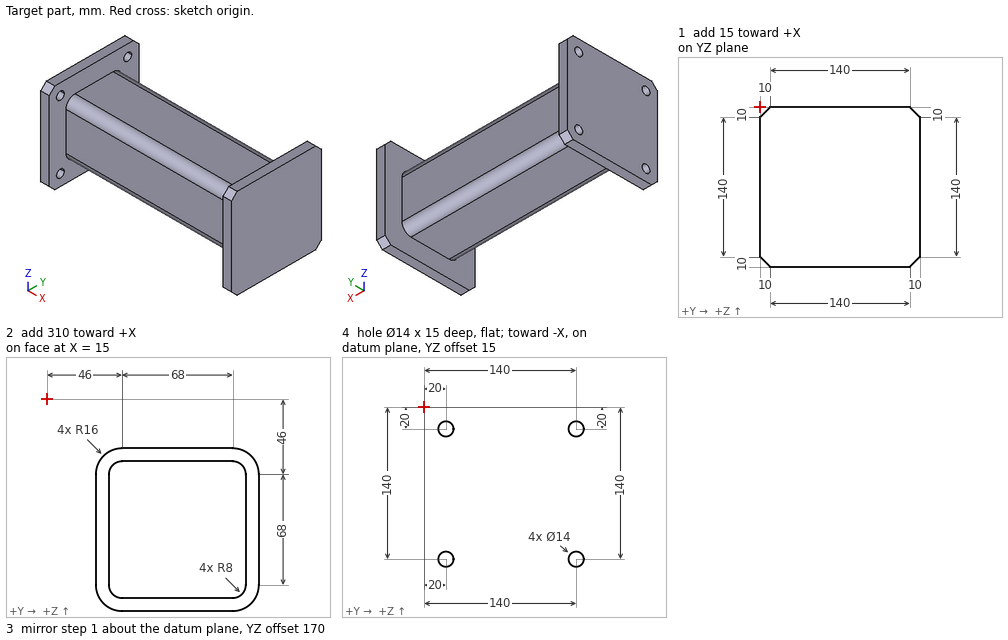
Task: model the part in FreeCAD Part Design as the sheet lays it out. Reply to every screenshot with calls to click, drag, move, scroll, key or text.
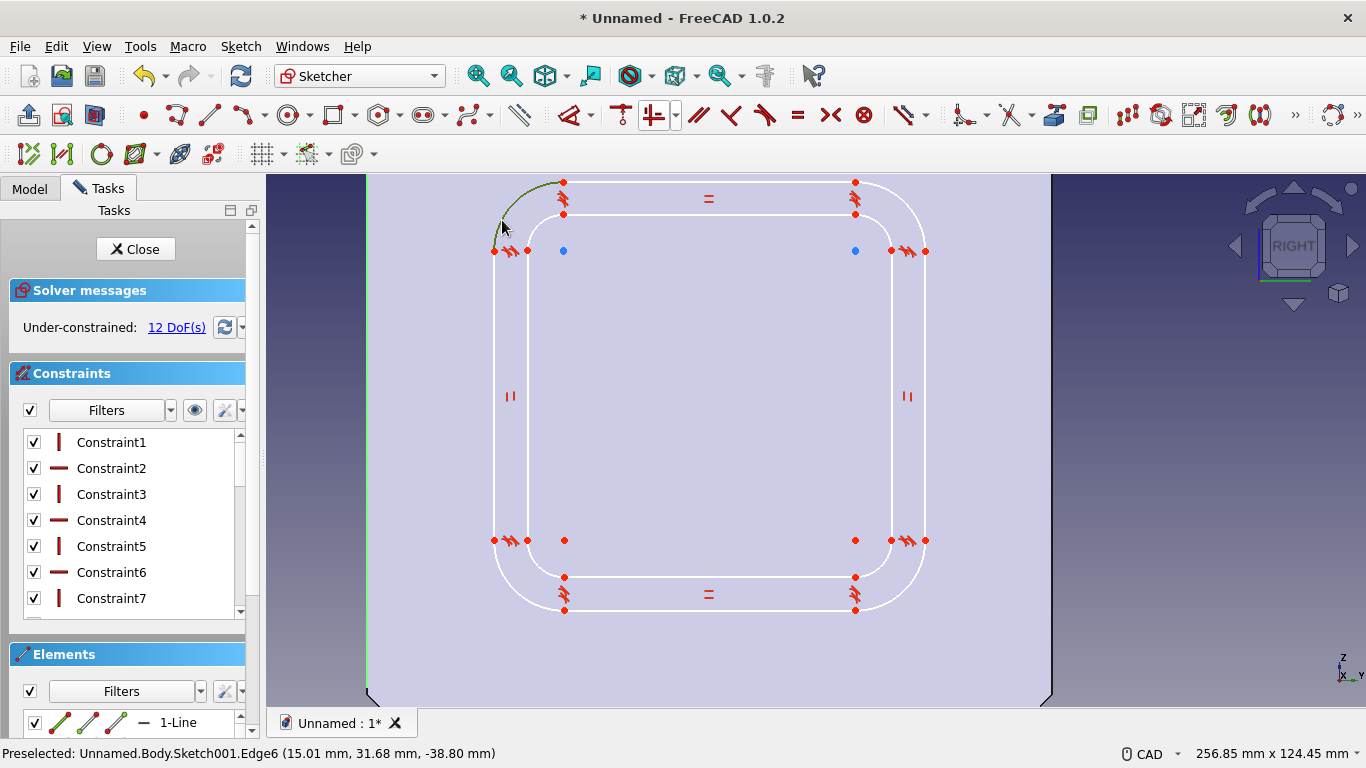
click(547, 219)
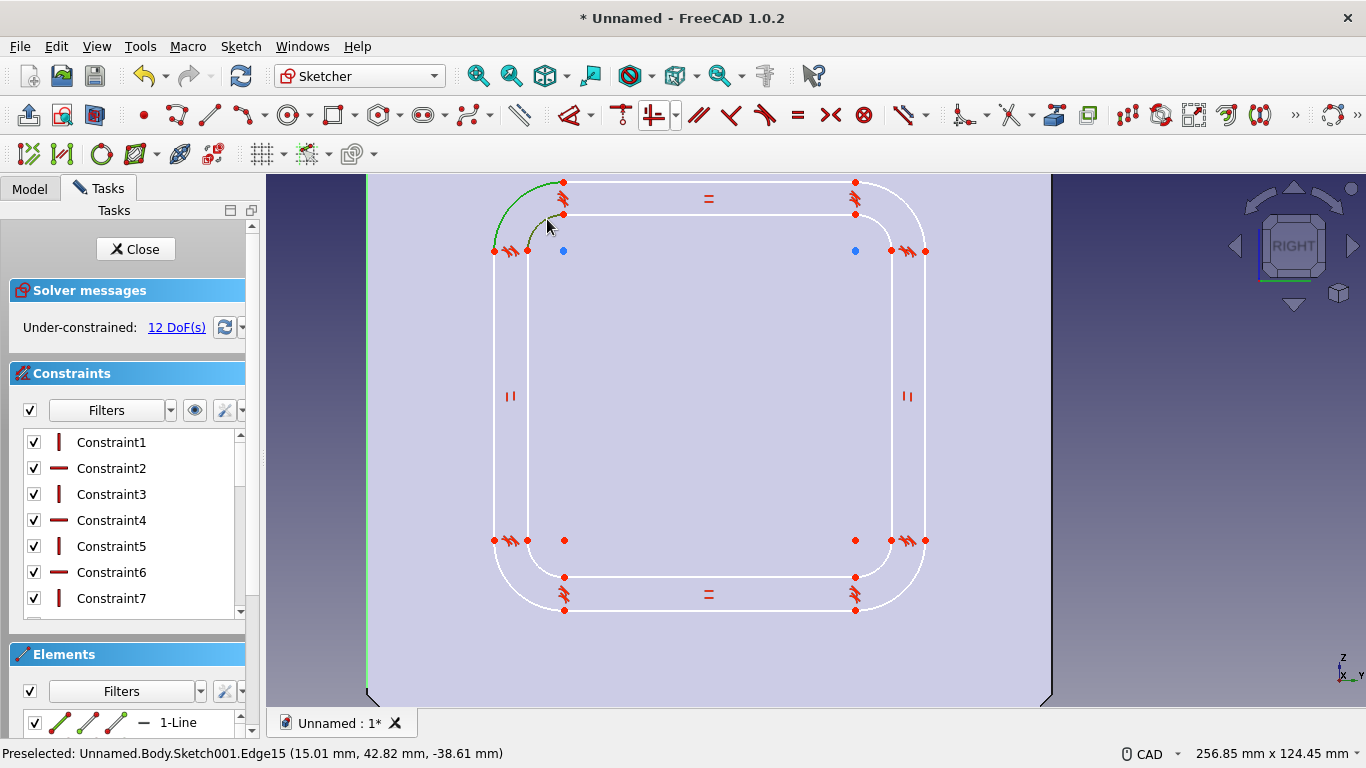
key(c)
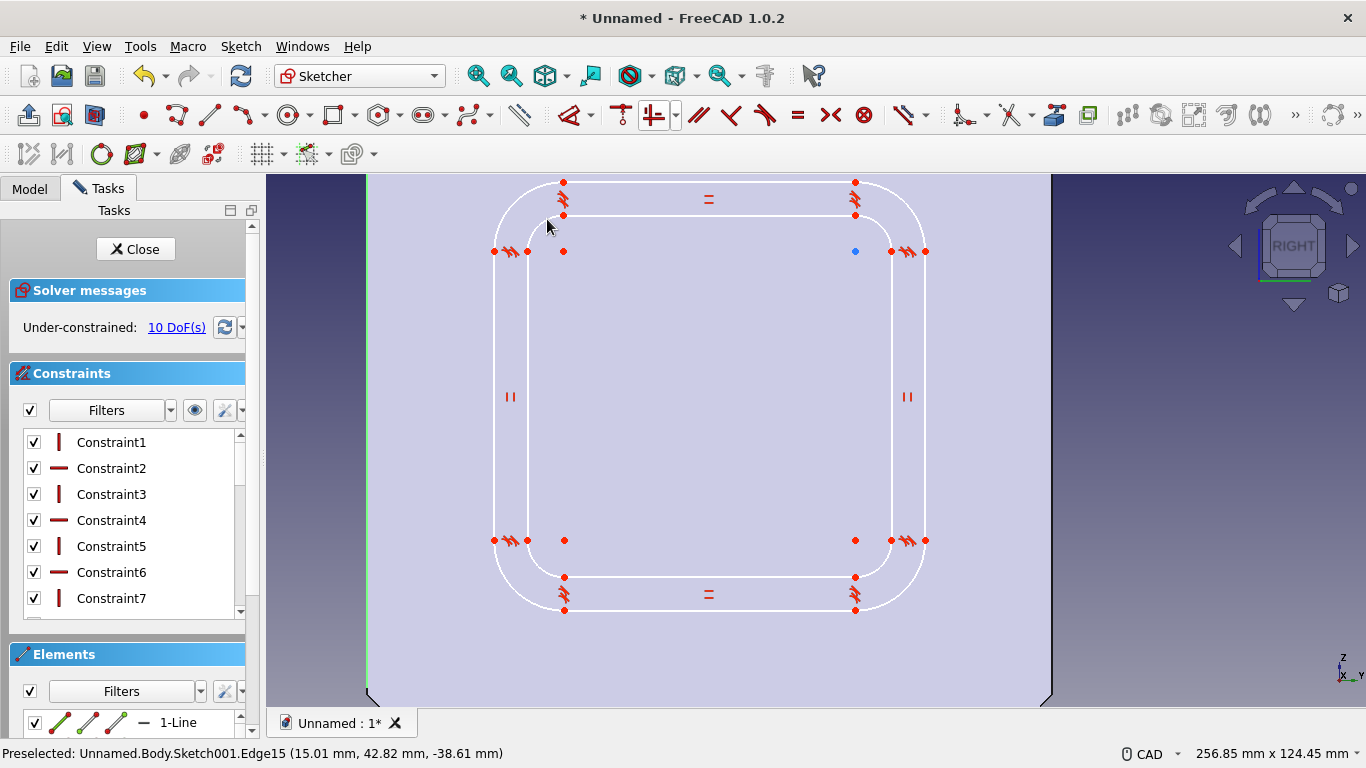
click(918, 220)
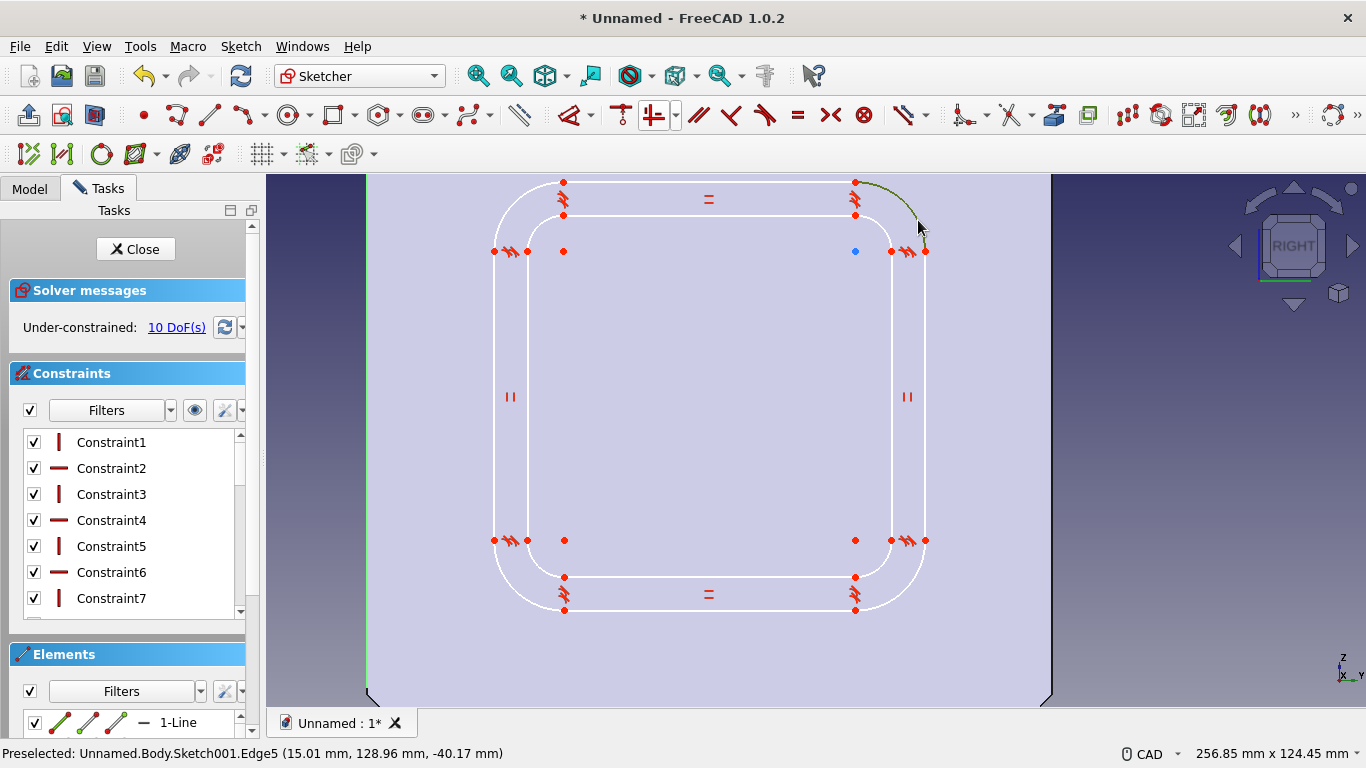
click(502, 220)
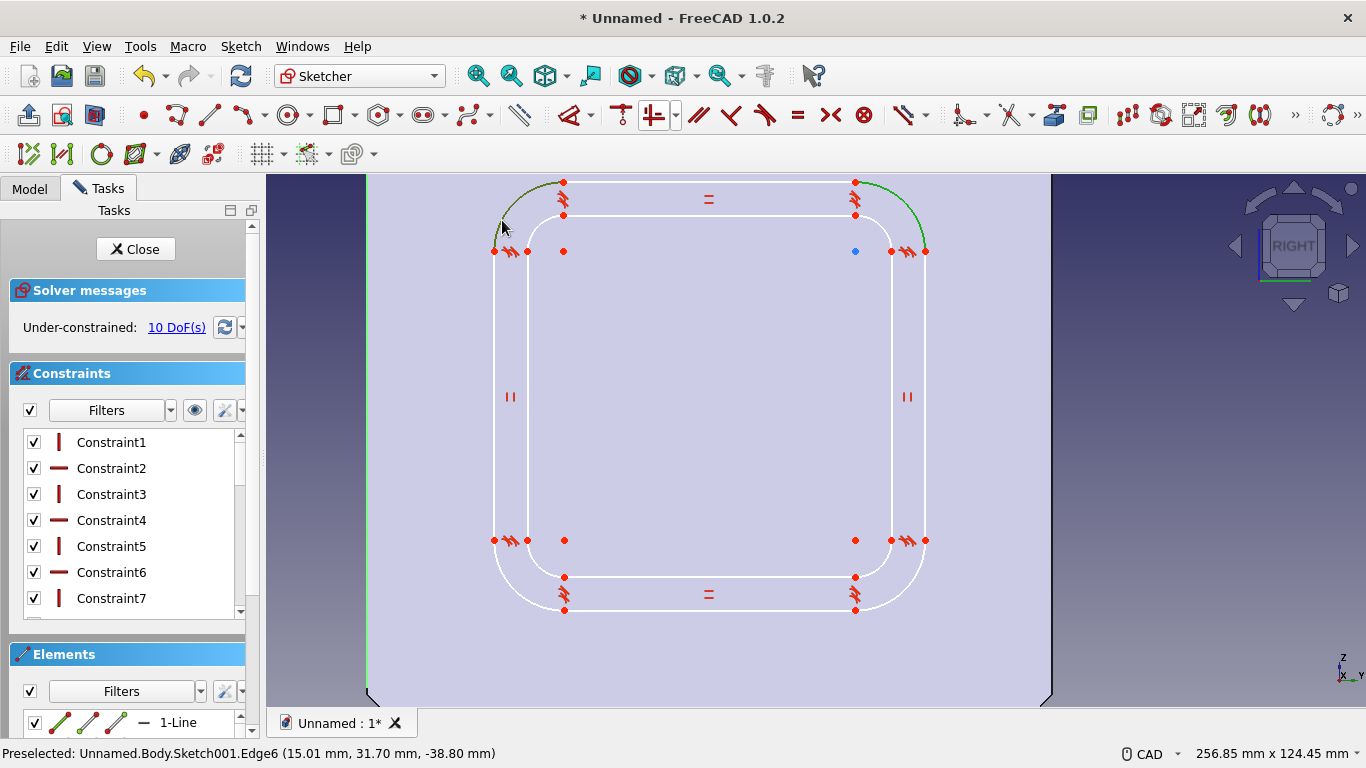
click(502, 573)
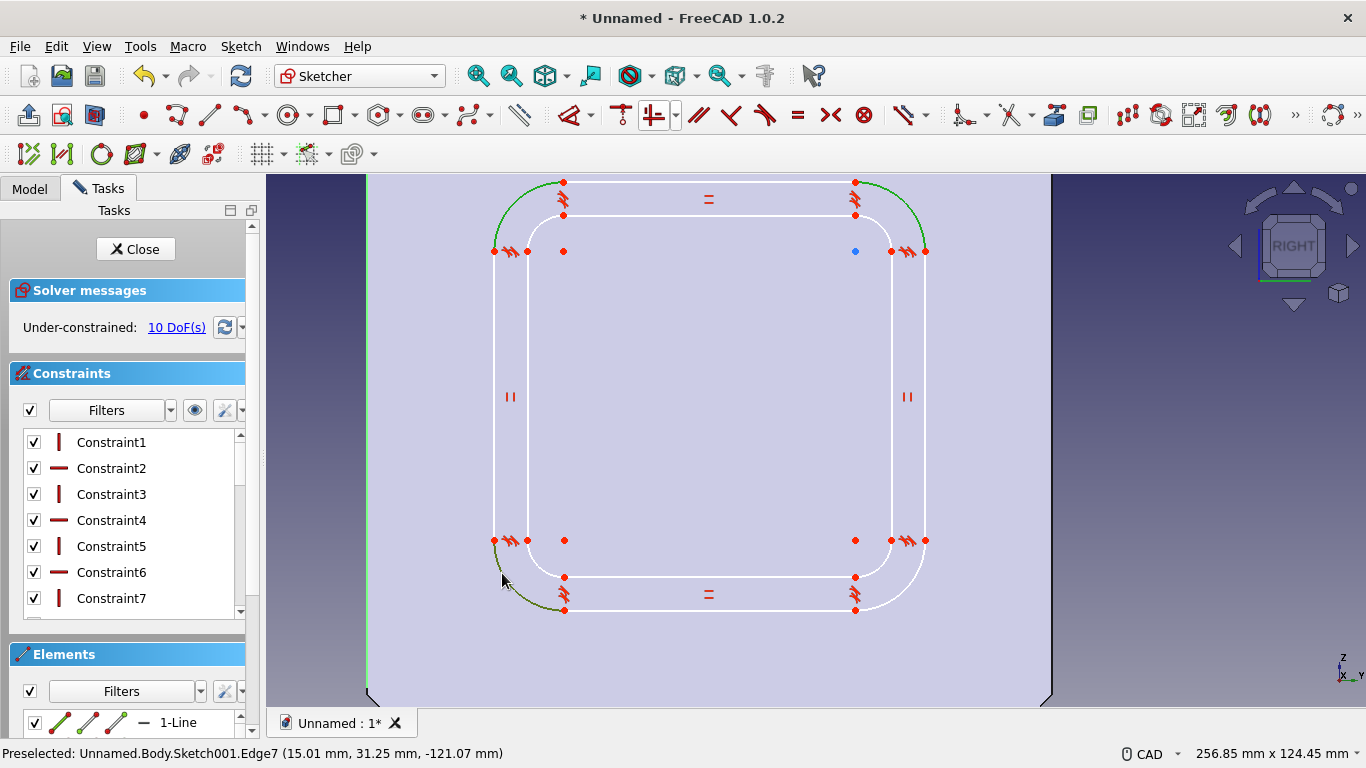
click(887, 603)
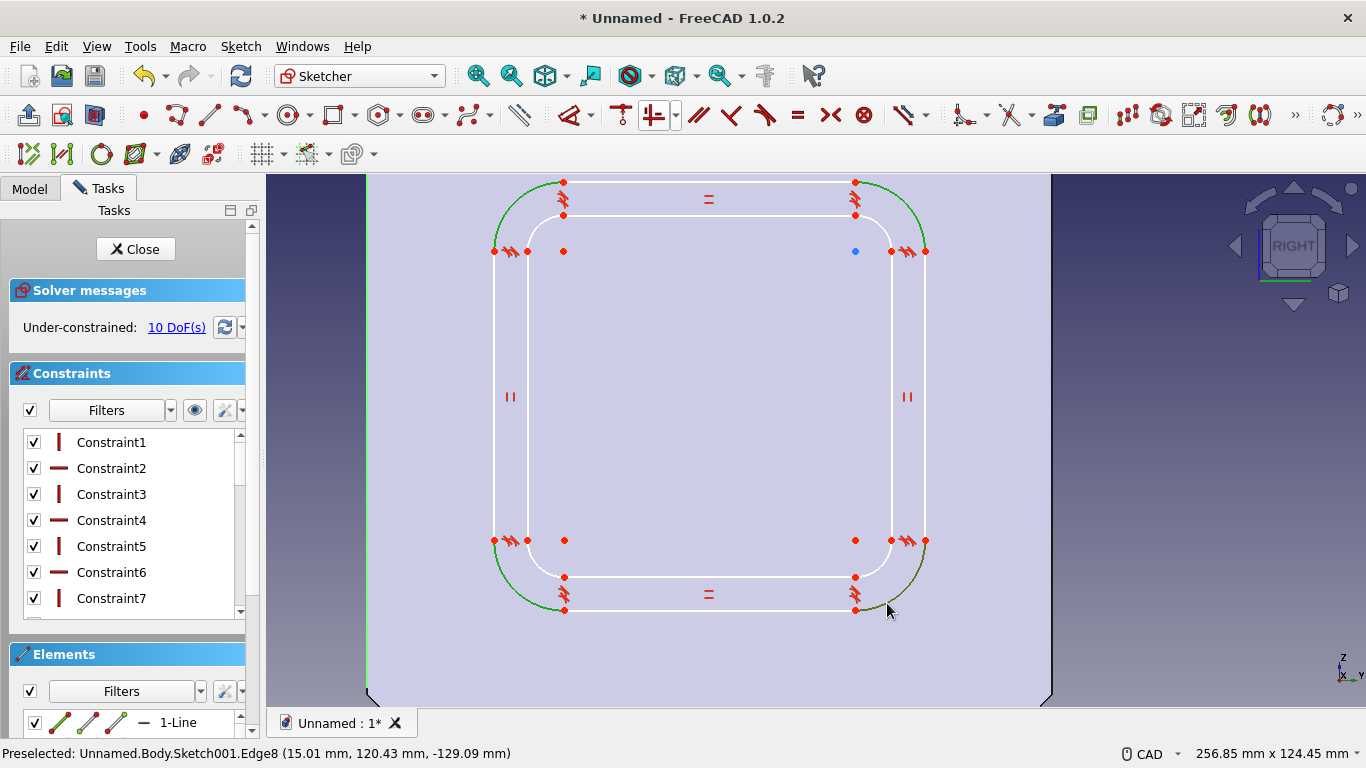
click(798, 116)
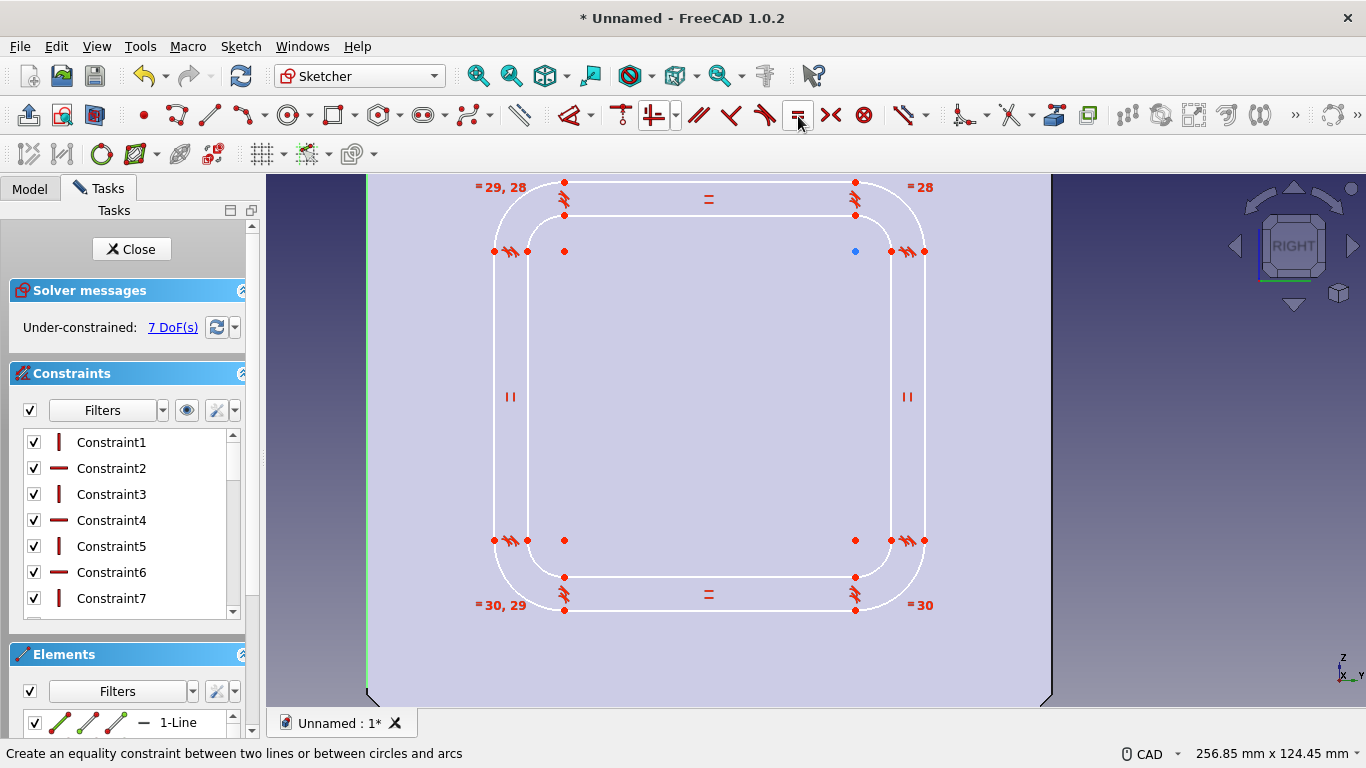
click(872, 573)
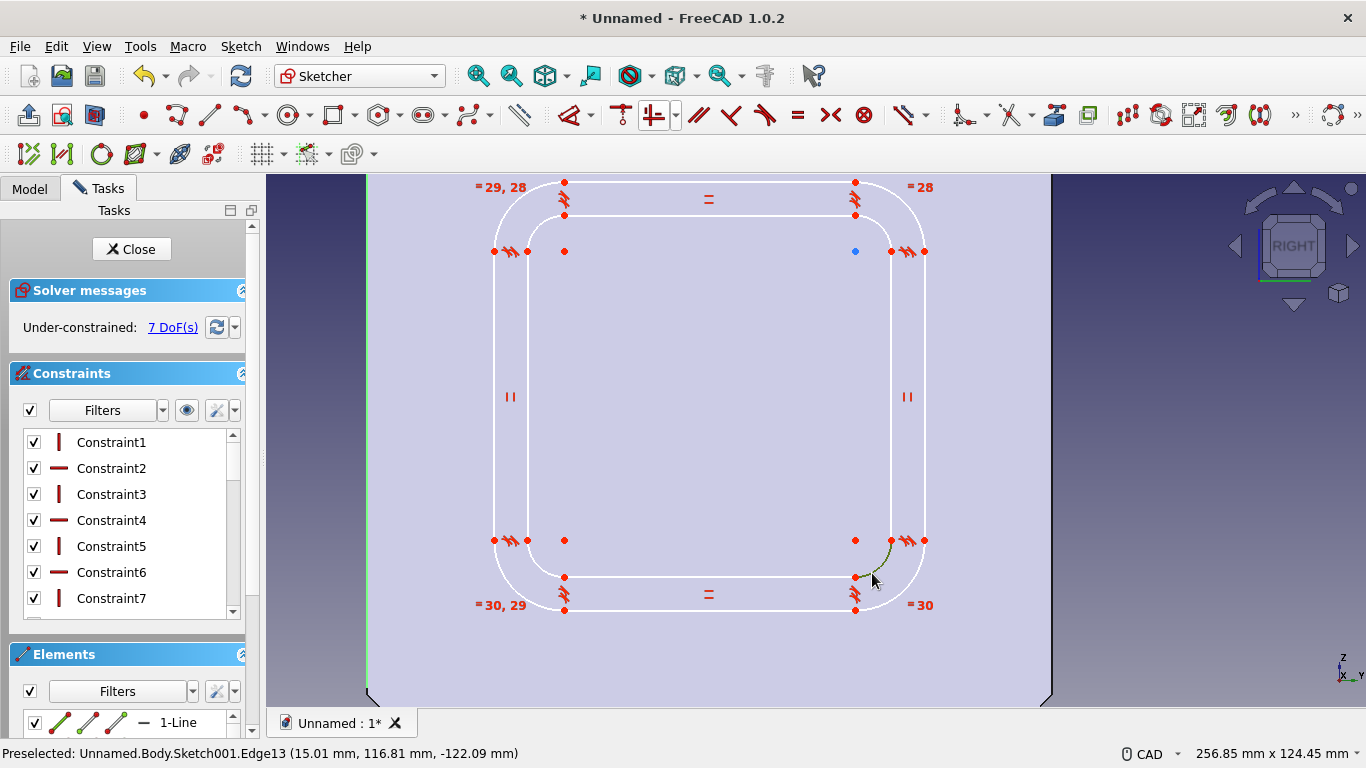
click(887, 235)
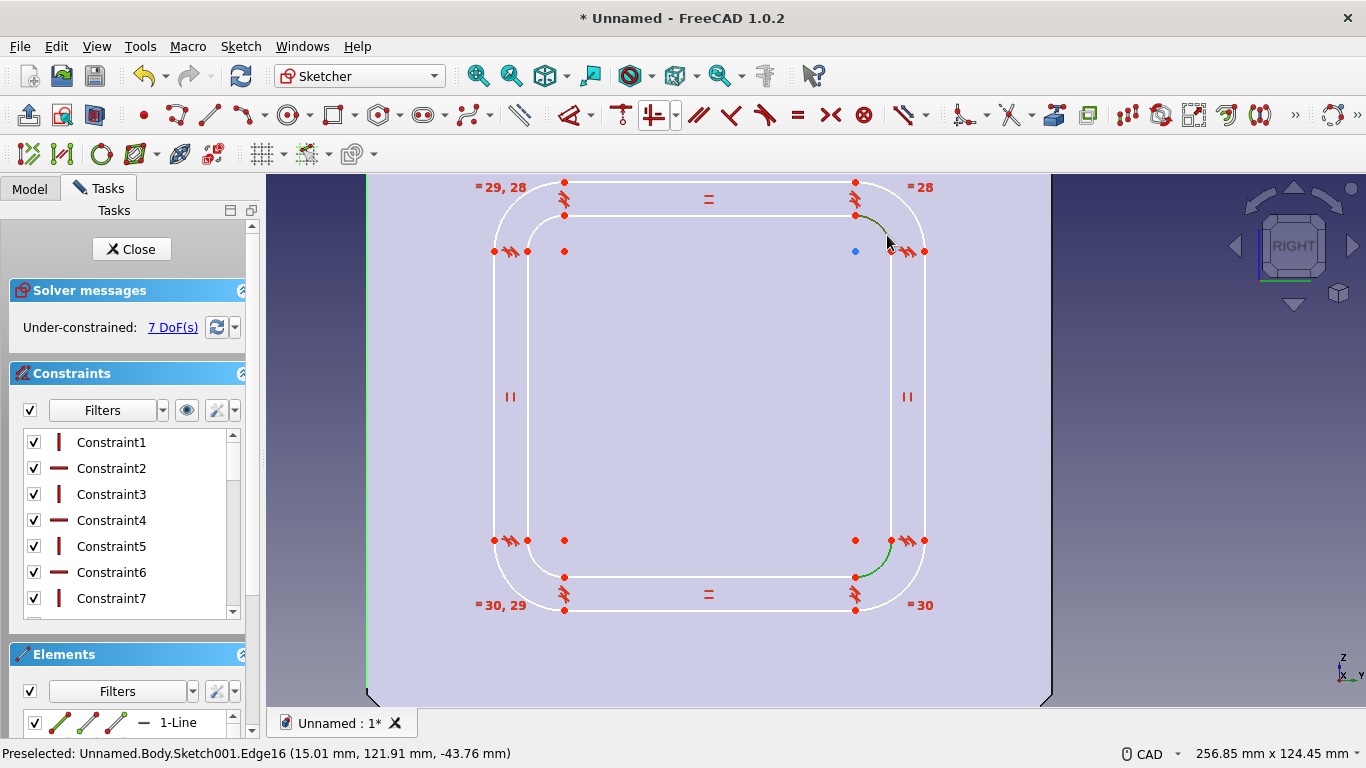
key(e)